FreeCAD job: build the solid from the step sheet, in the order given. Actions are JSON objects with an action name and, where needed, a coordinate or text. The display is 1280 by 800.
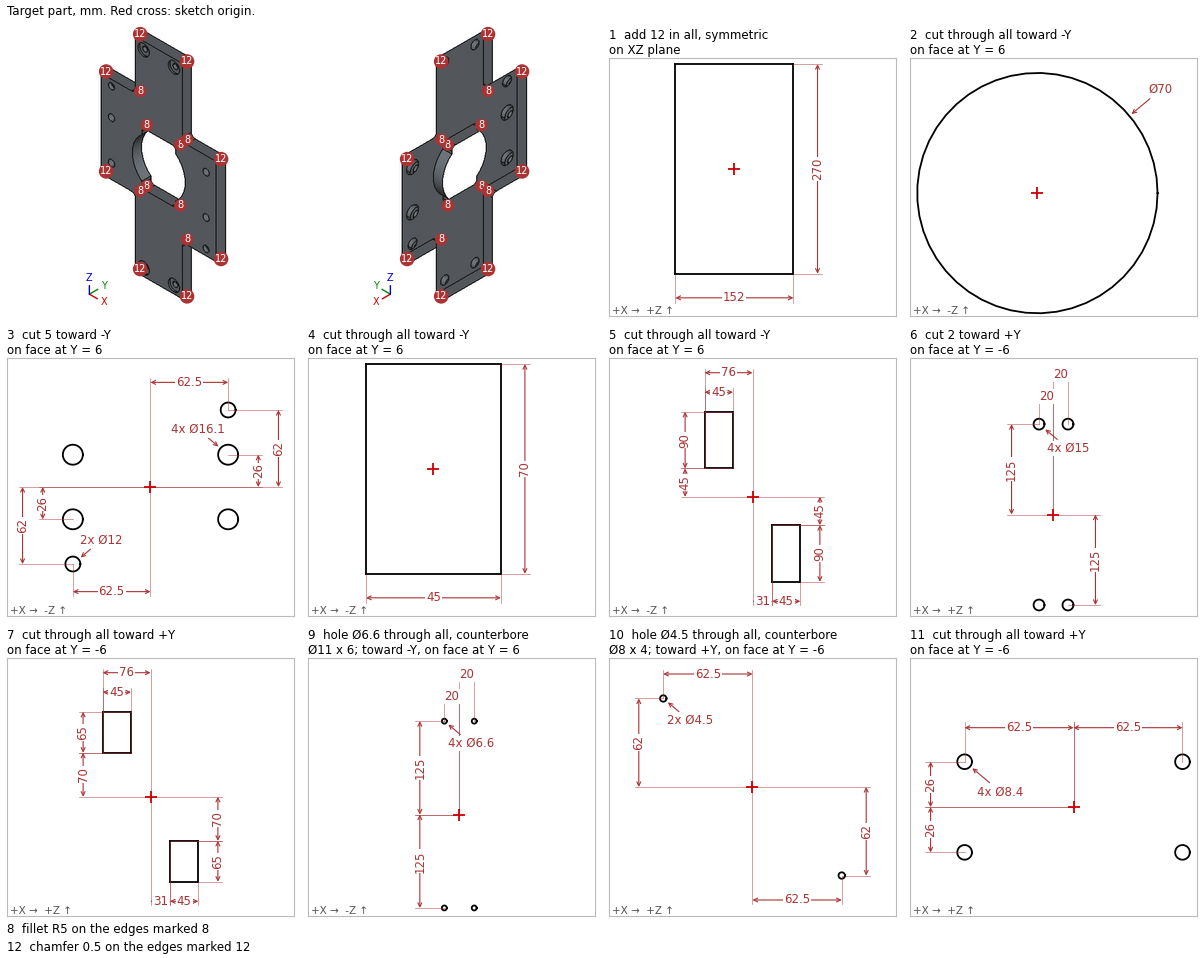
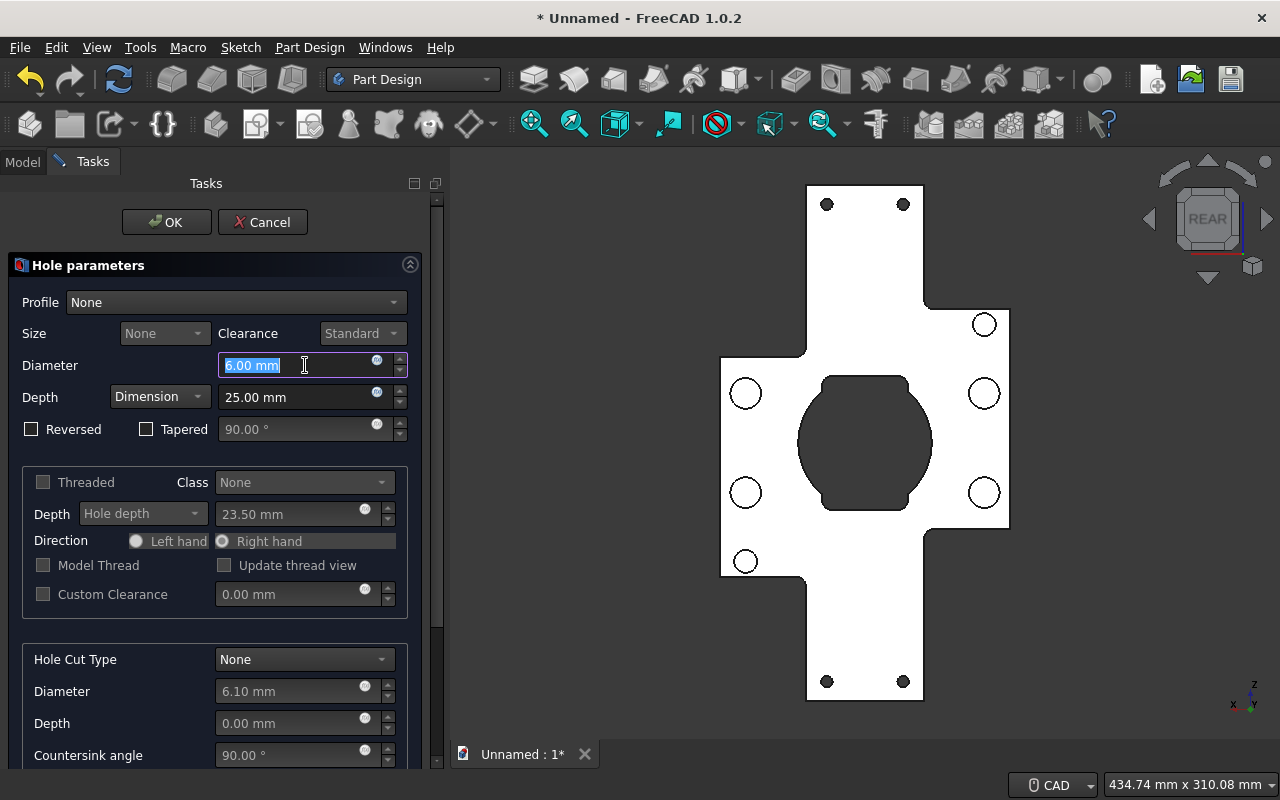
{"action": "type", "text": "6.6"}
{"action": "key", "text": "Tab"}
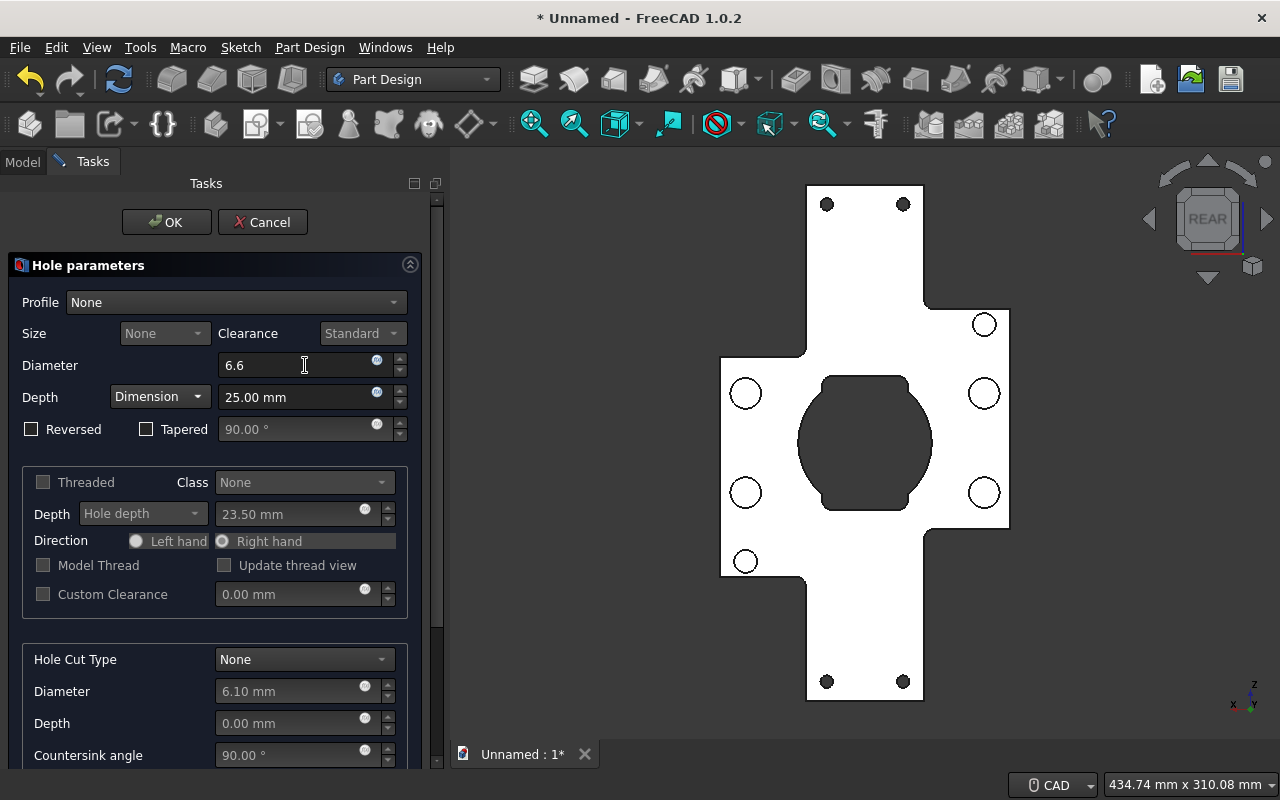
{"action": "left_click", "coordinate": [161, 396]}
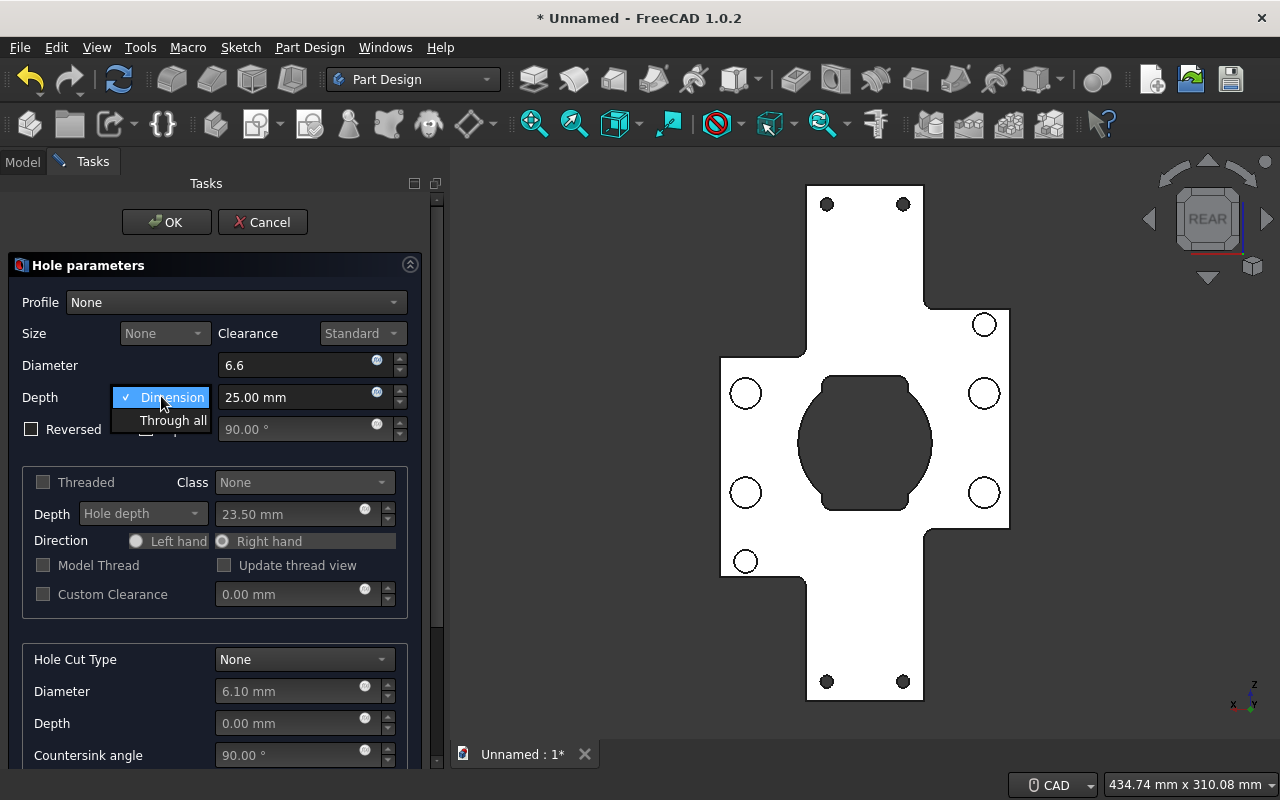
{"action": "left_click", "coordinate": [160, 420]}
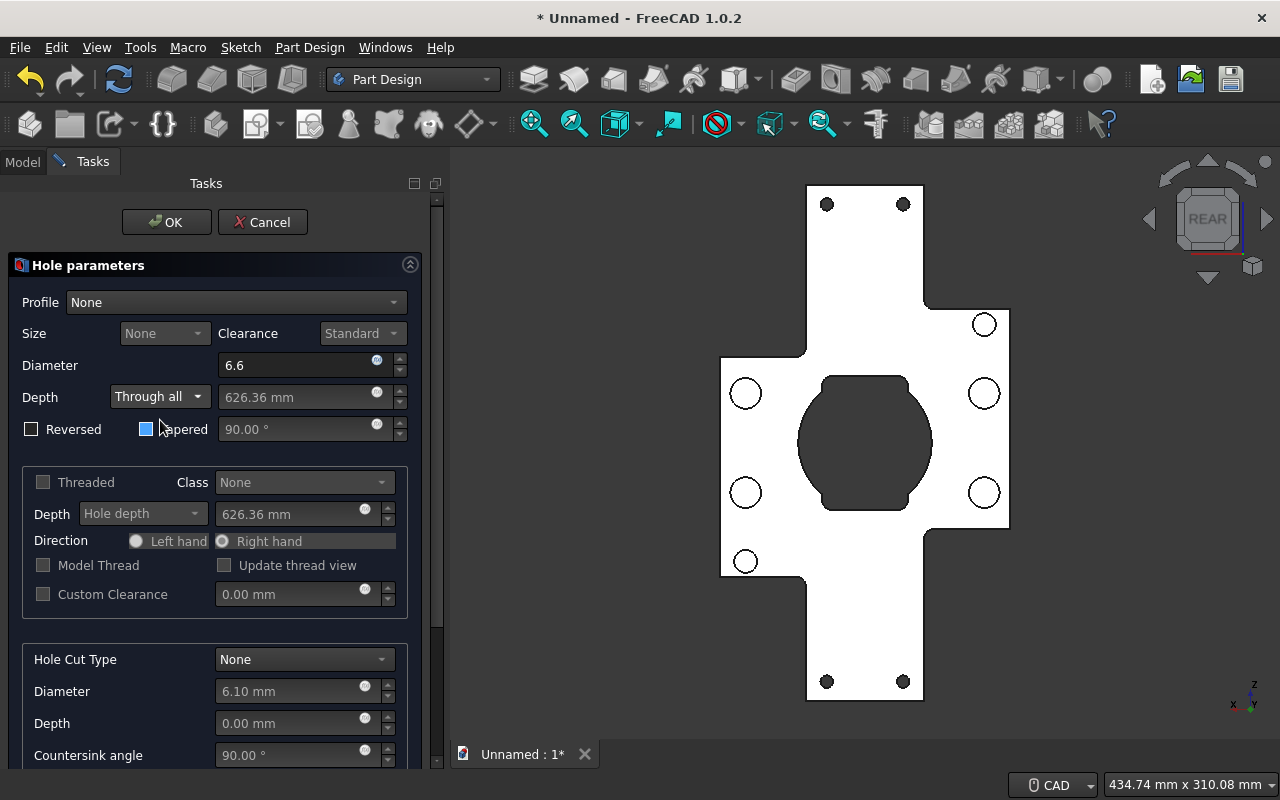
{"action": "left_click", "coordinate": [306, 660]}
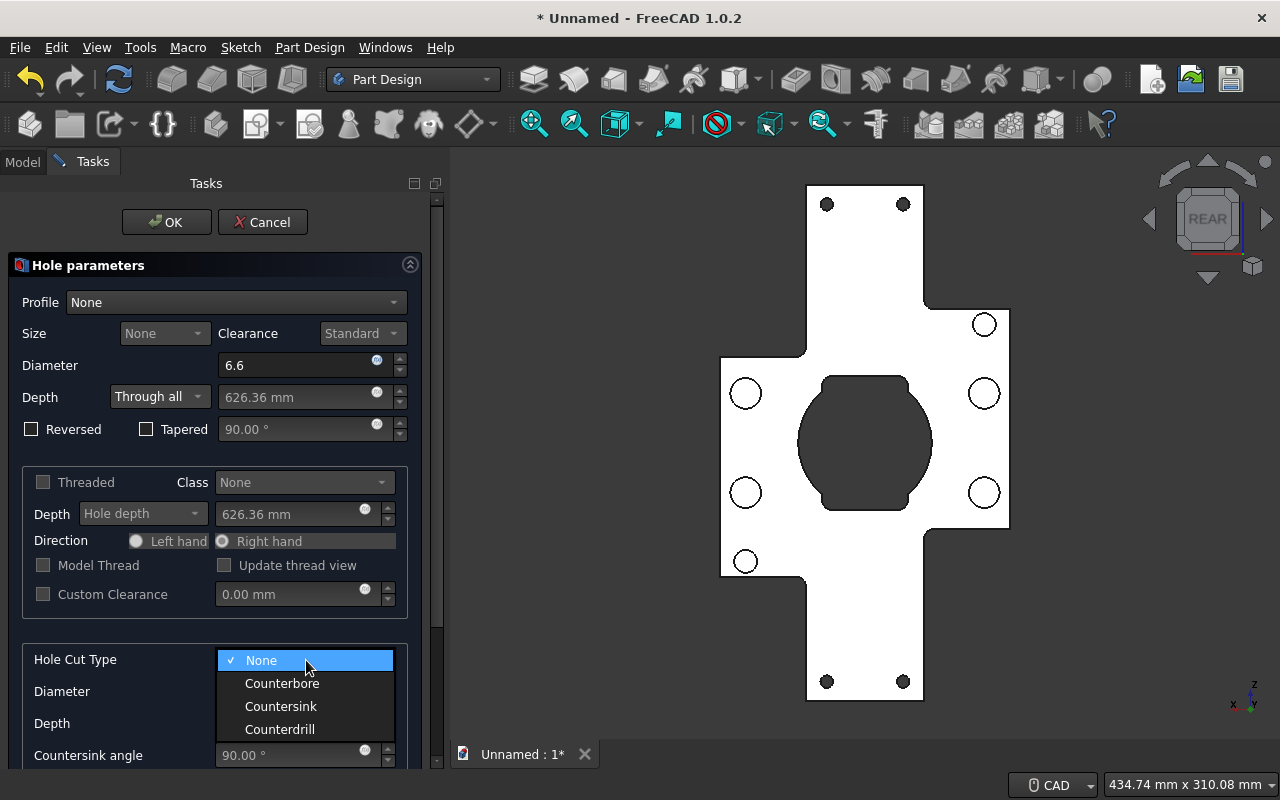
{"action": "left_click", "coordinate": [304, 684]}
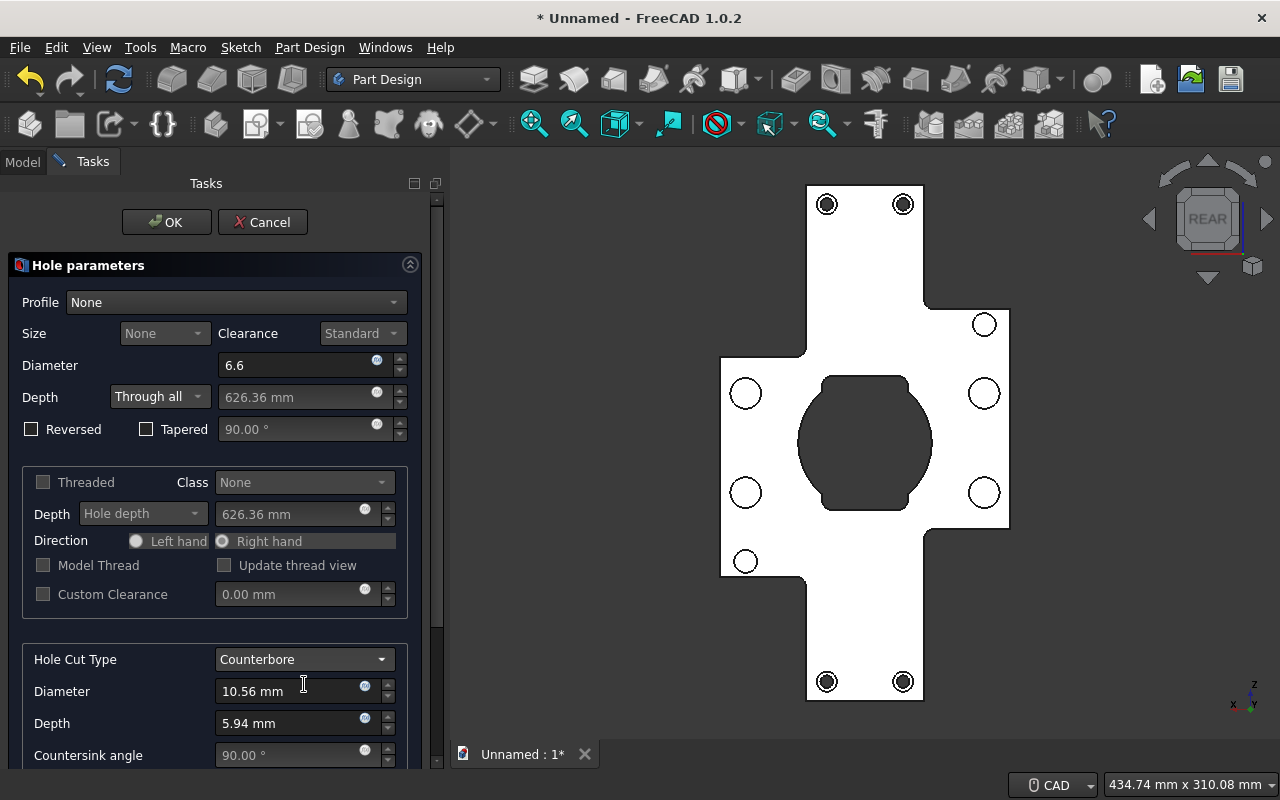
{"action": "triple_click", "coordinate": [298, 691]}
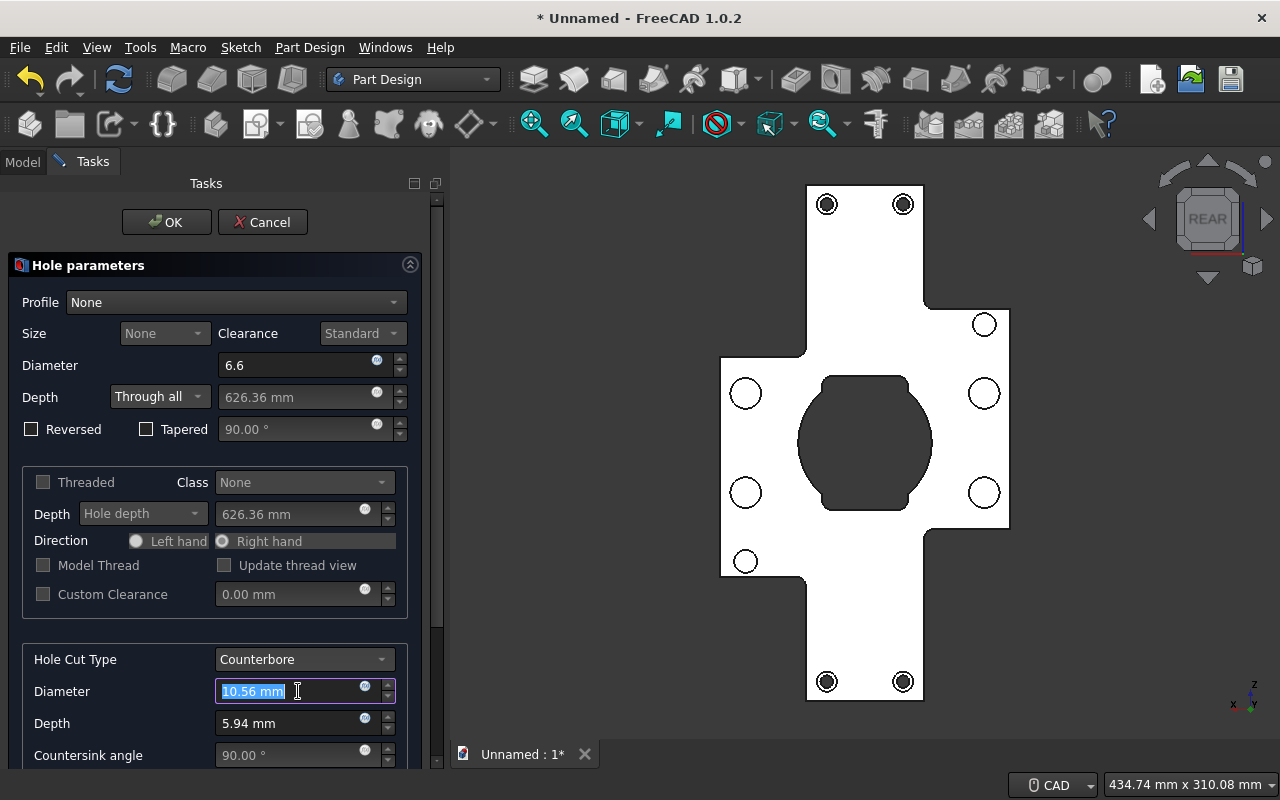
{"action": "type", "text": "11"}
{"action": "key", "text": "Tab"}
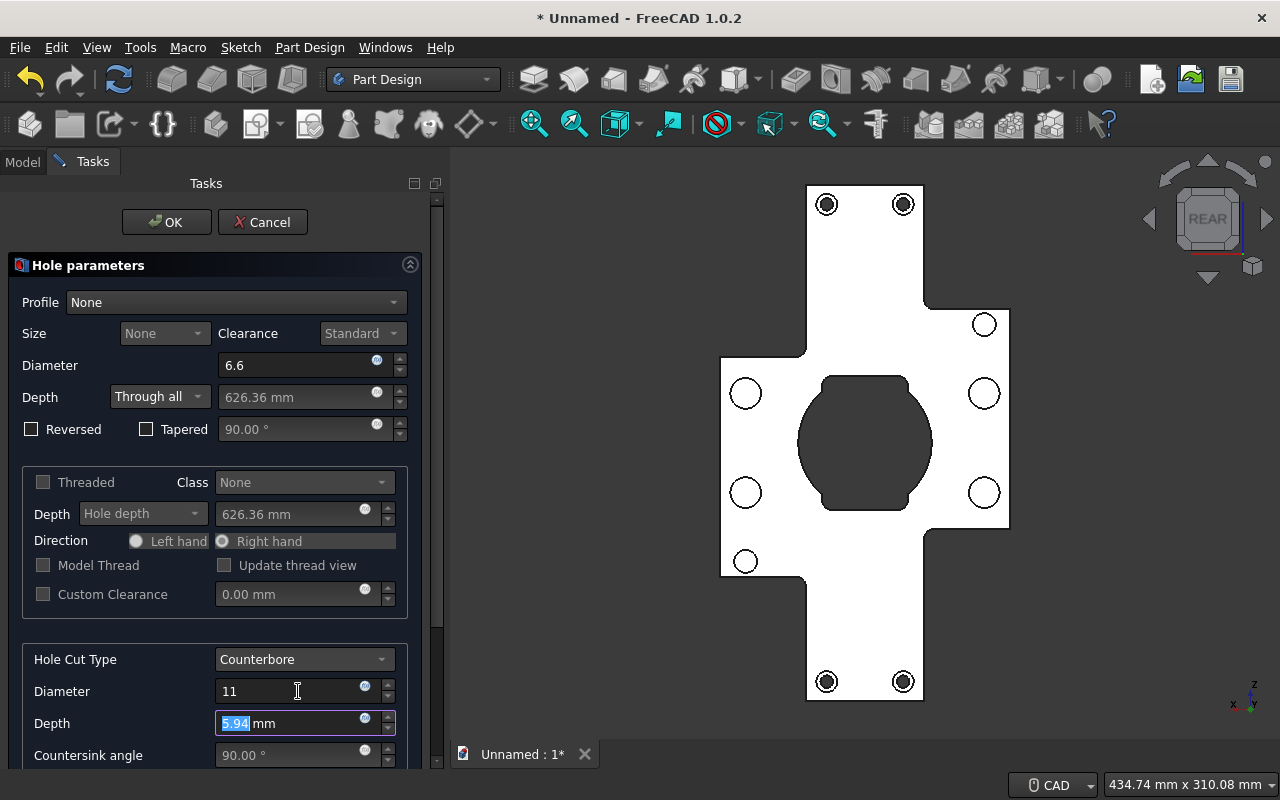
{"action": "type", "text": "6"}
{"action": "key", "text": "Tab"}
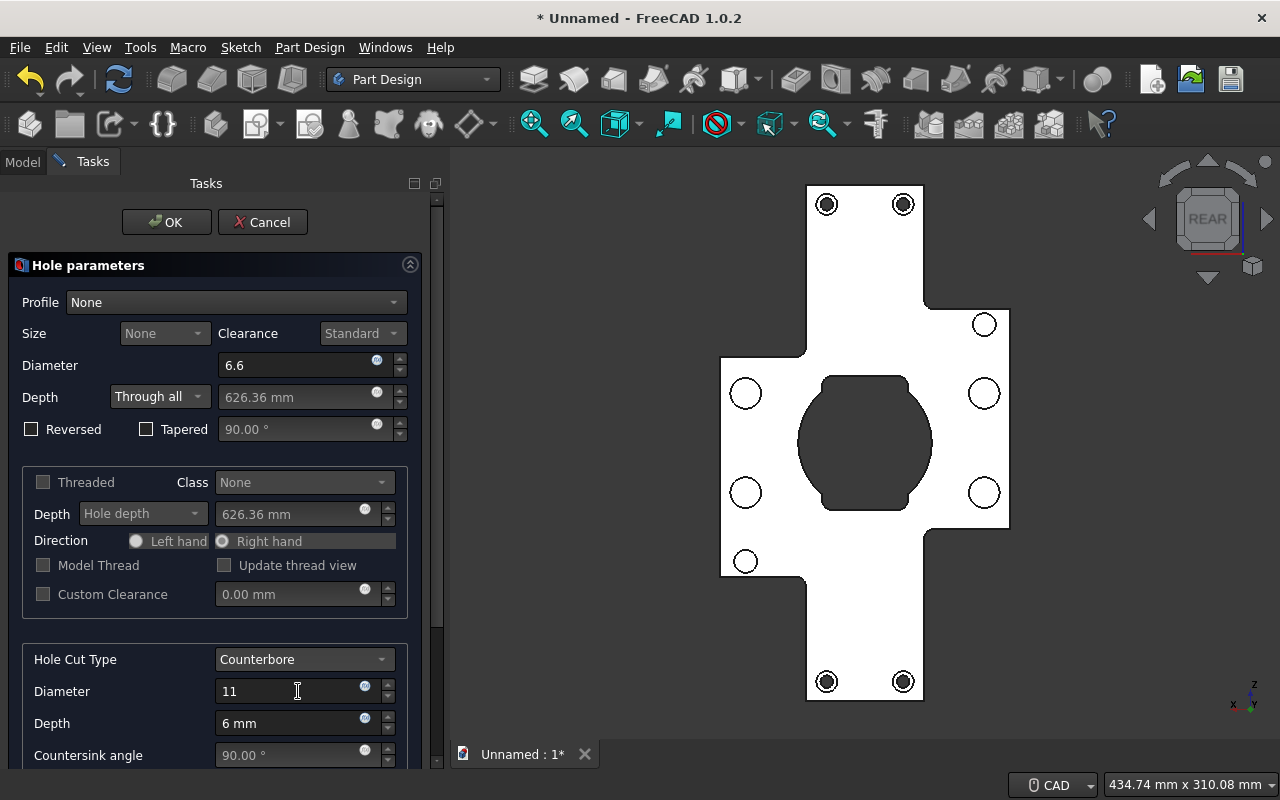
{"action": "left_click", "coordinate": [167, 222]}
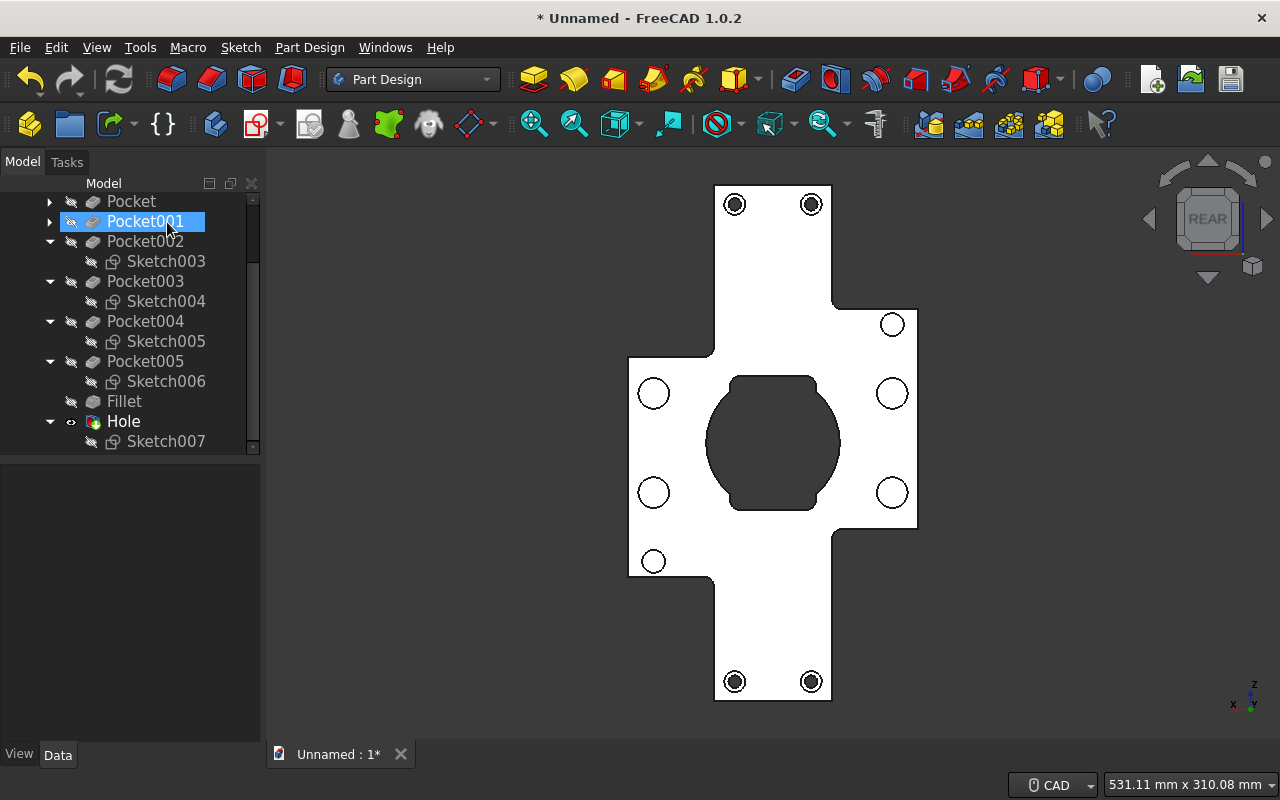
{"action": "key", "text": "0"}